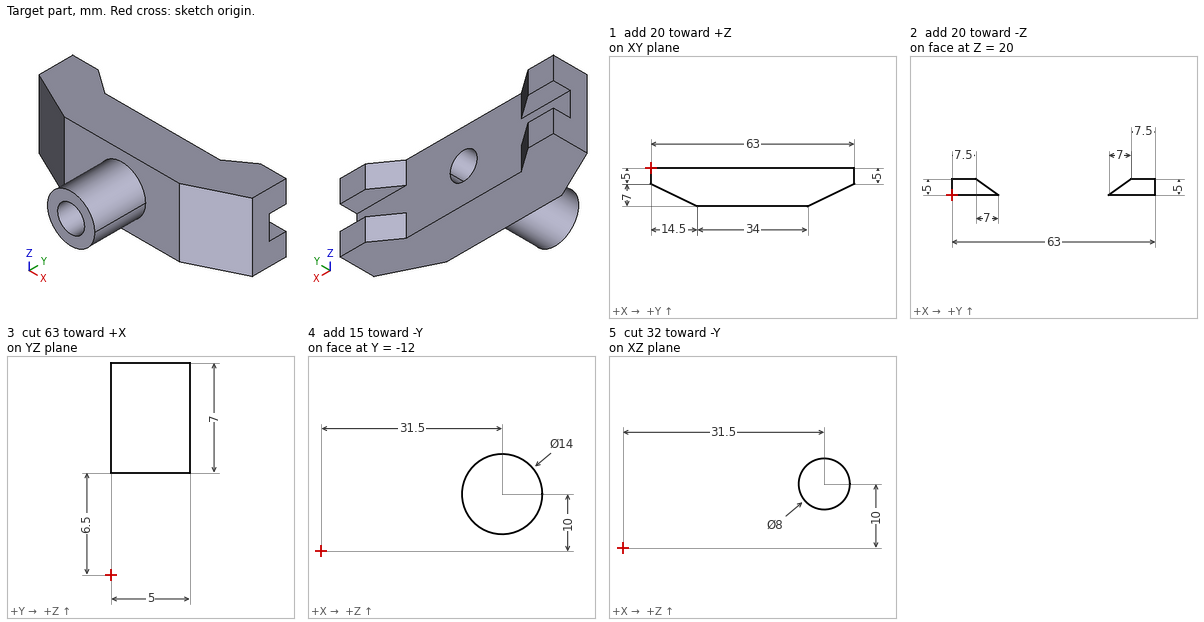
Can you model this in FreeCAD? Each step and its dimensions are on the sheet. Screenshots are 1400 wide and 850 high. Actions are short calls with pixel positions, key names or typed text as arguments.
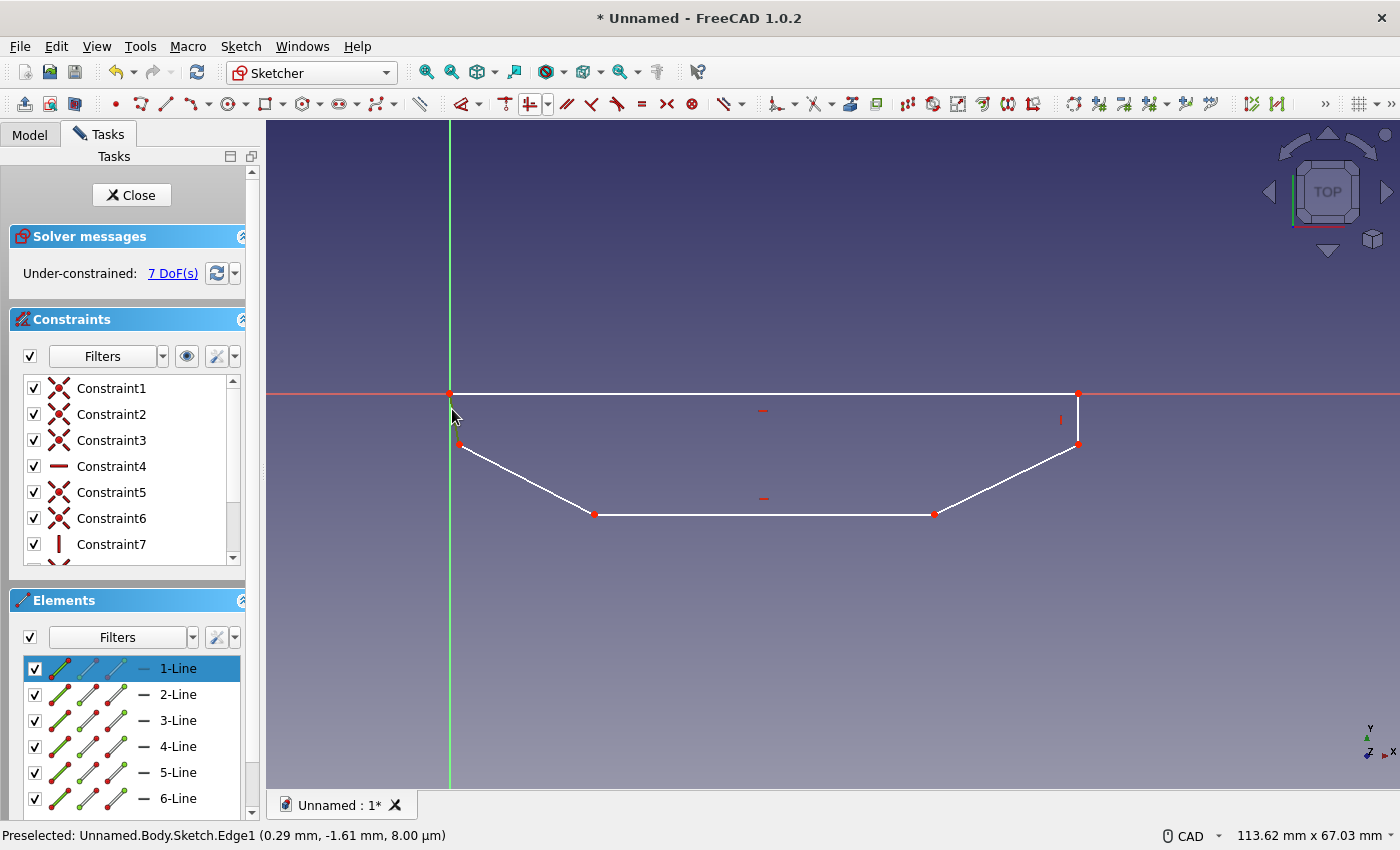
click(548, 104)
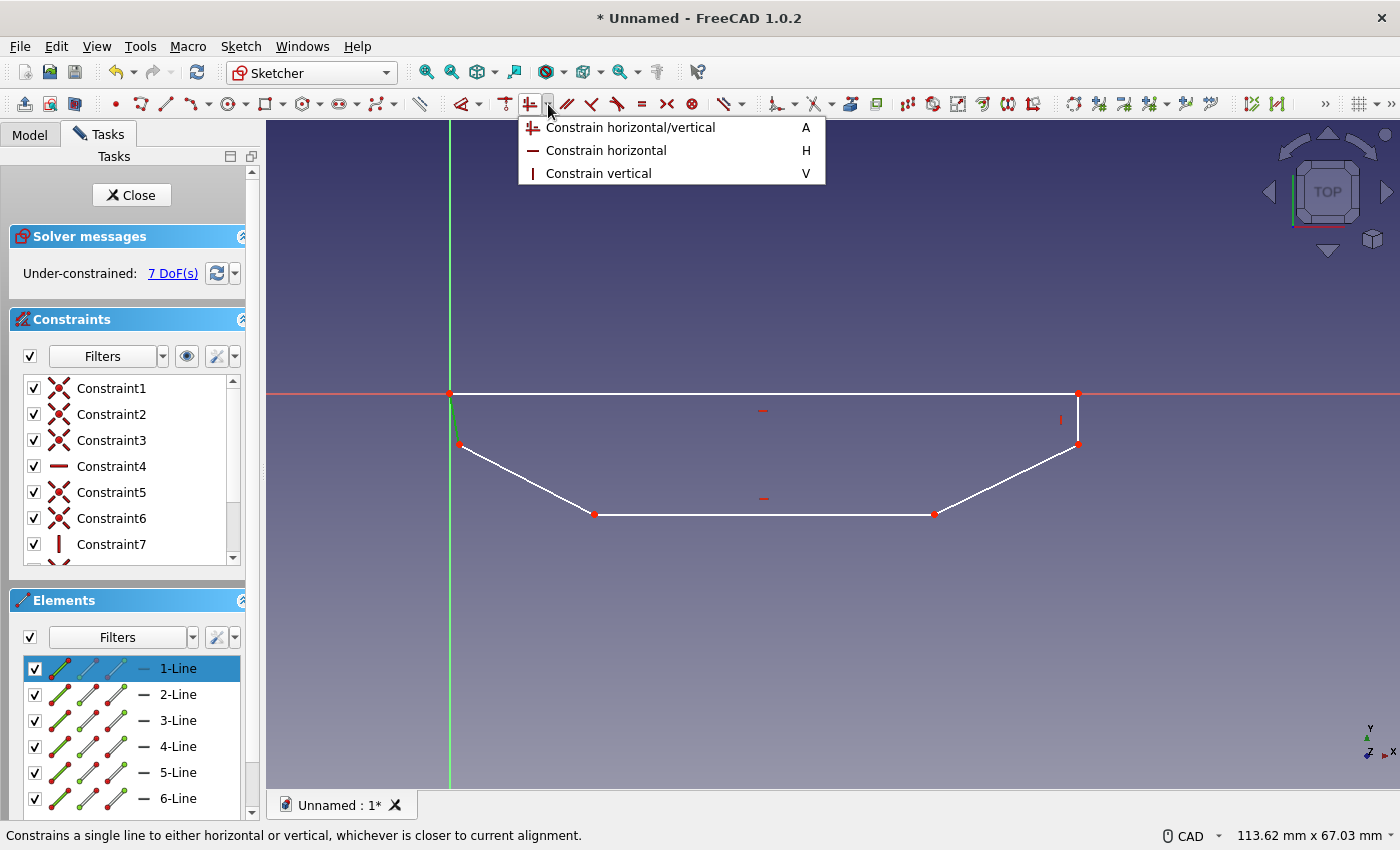
click(672, 174)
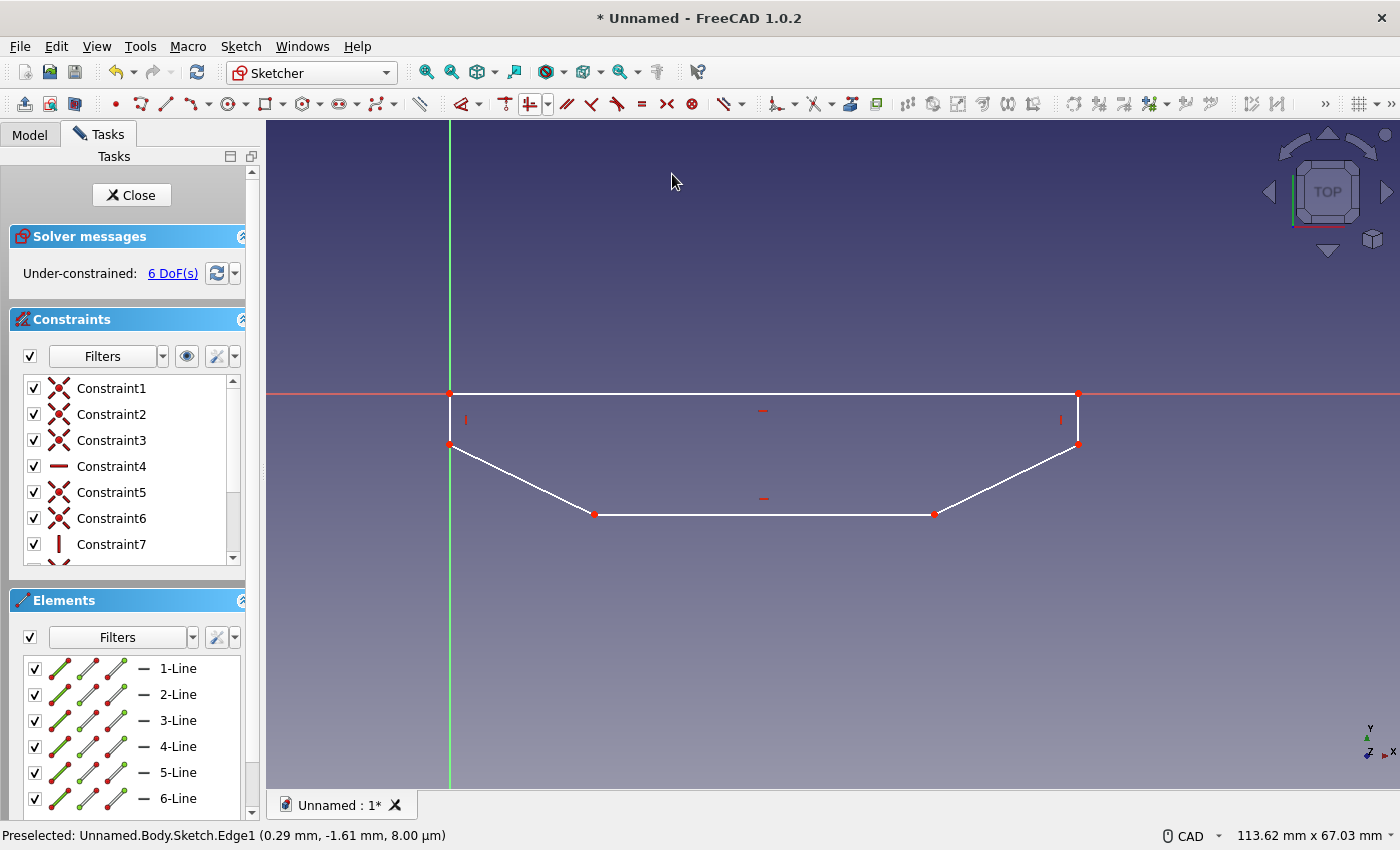
click(460, 104)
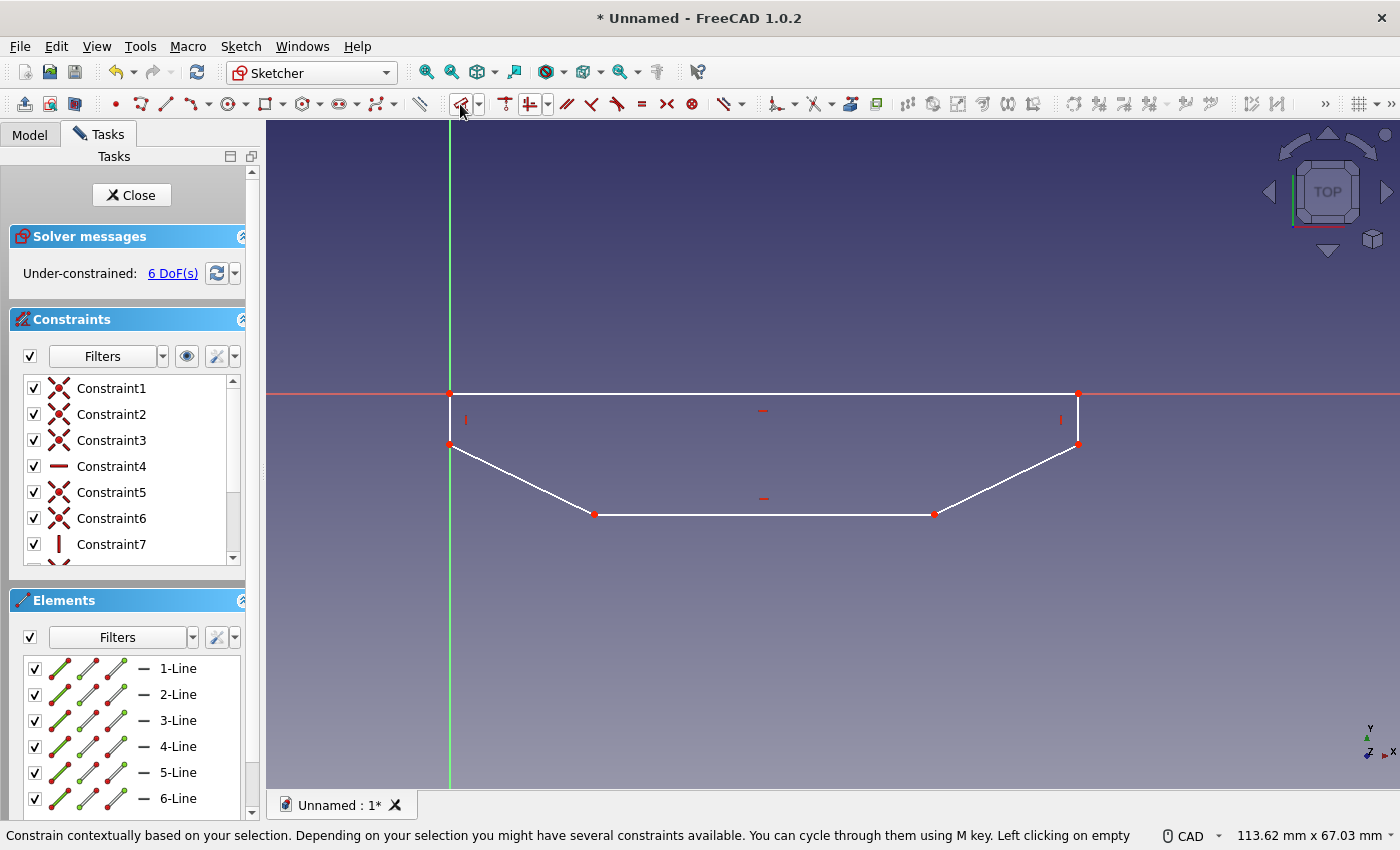
click(450, 409)
click(416, 419)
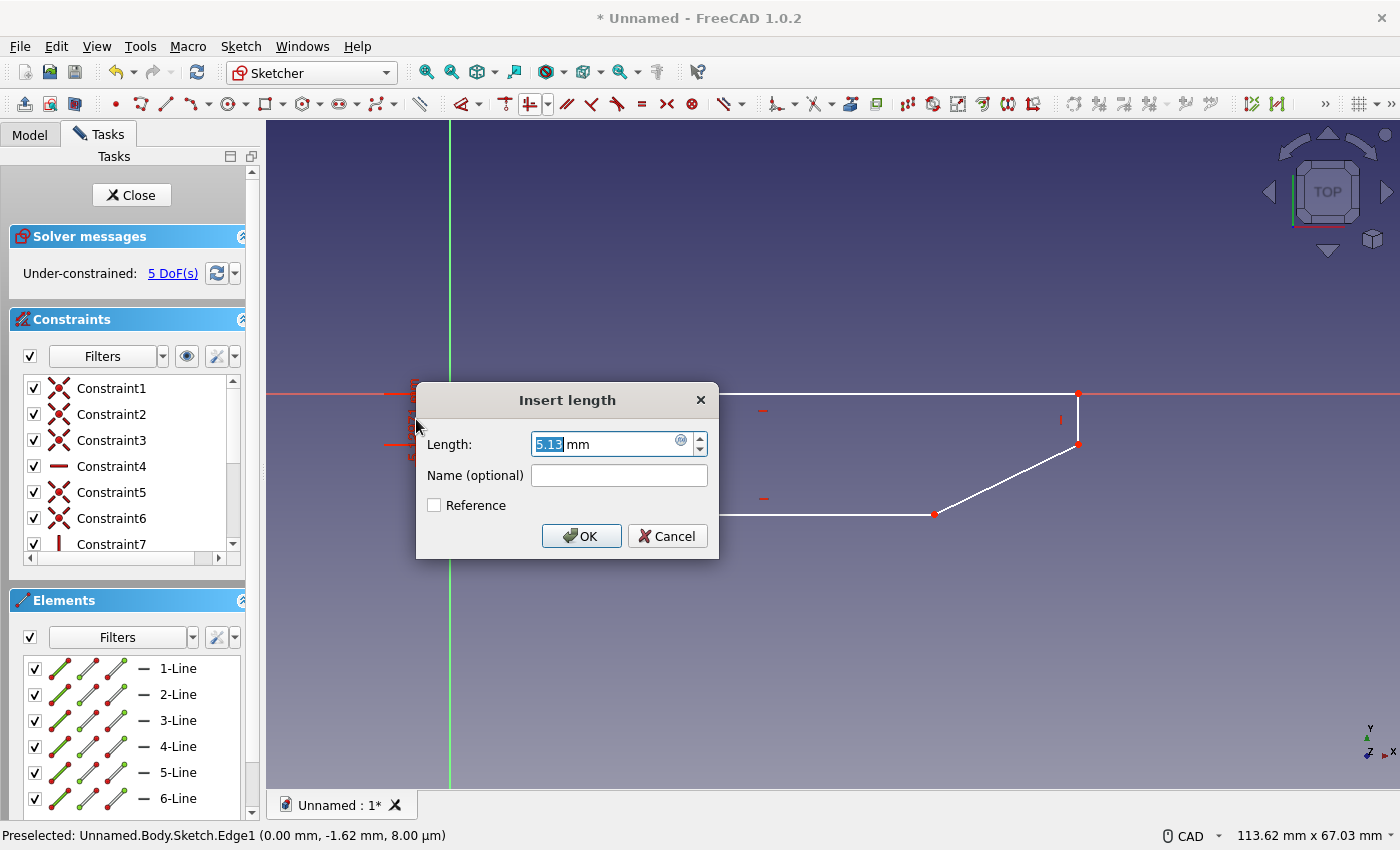
text(5)
key(Return)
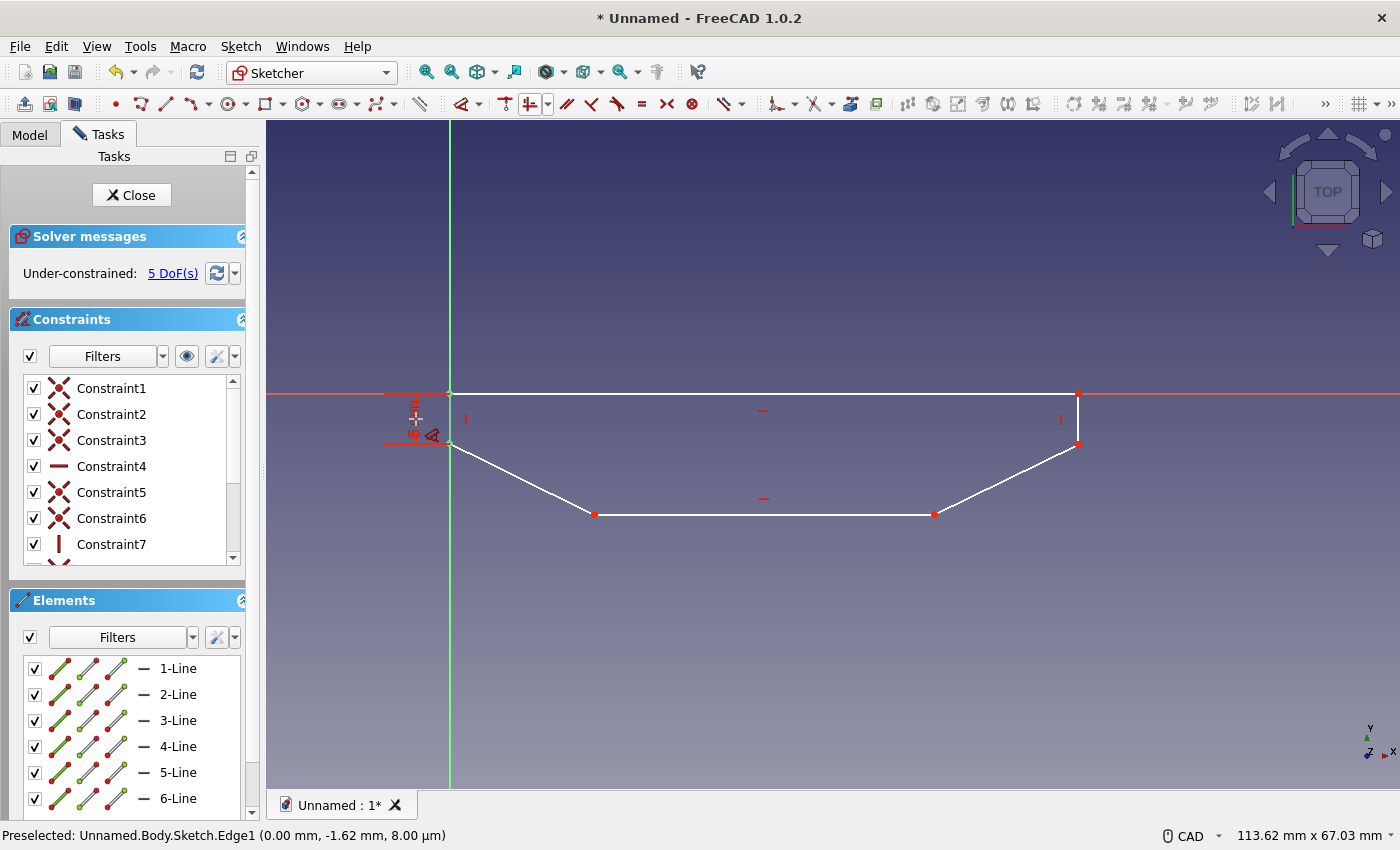
click(1078, 430)
click(1112, 419)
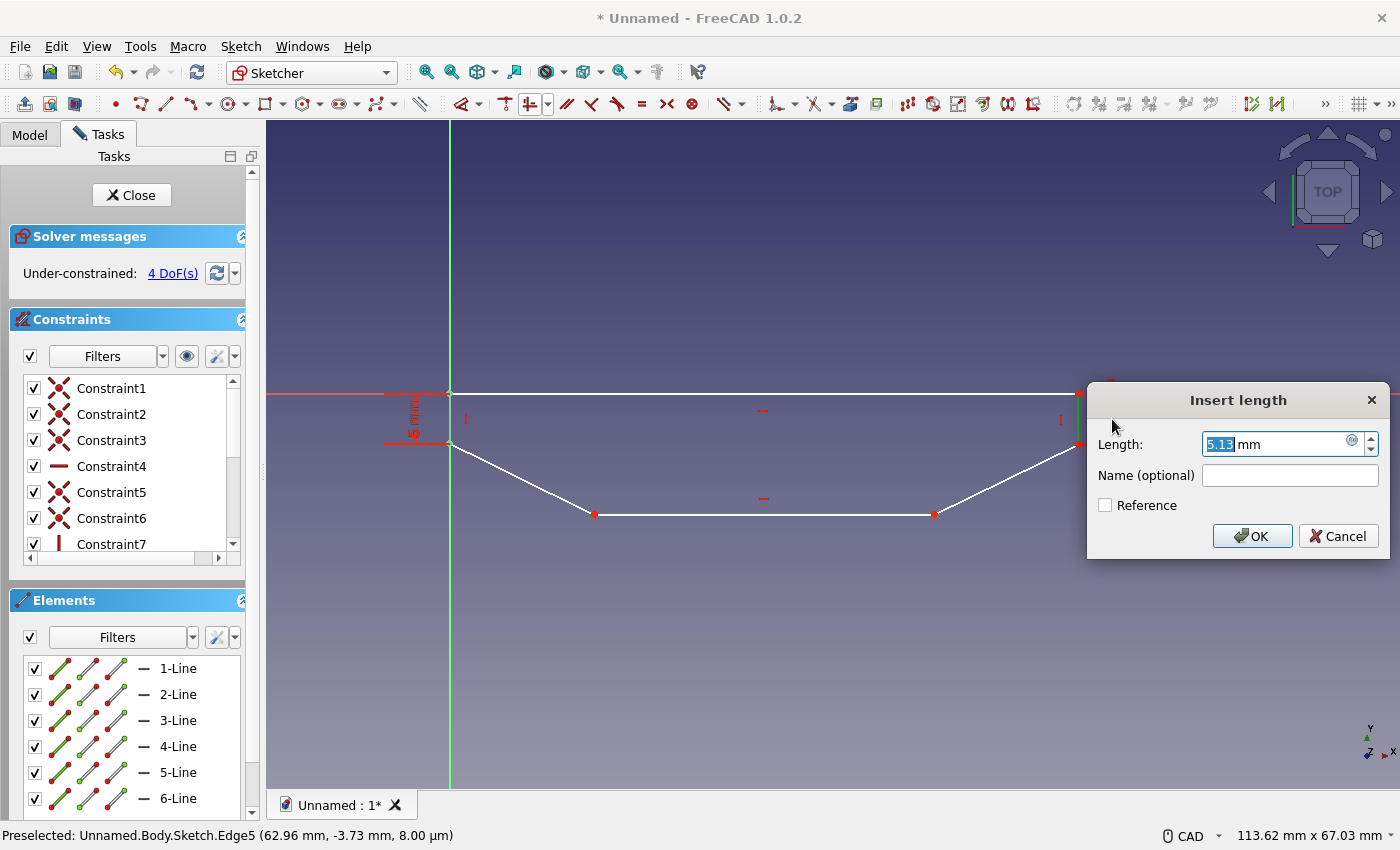
text(5)
key(Return)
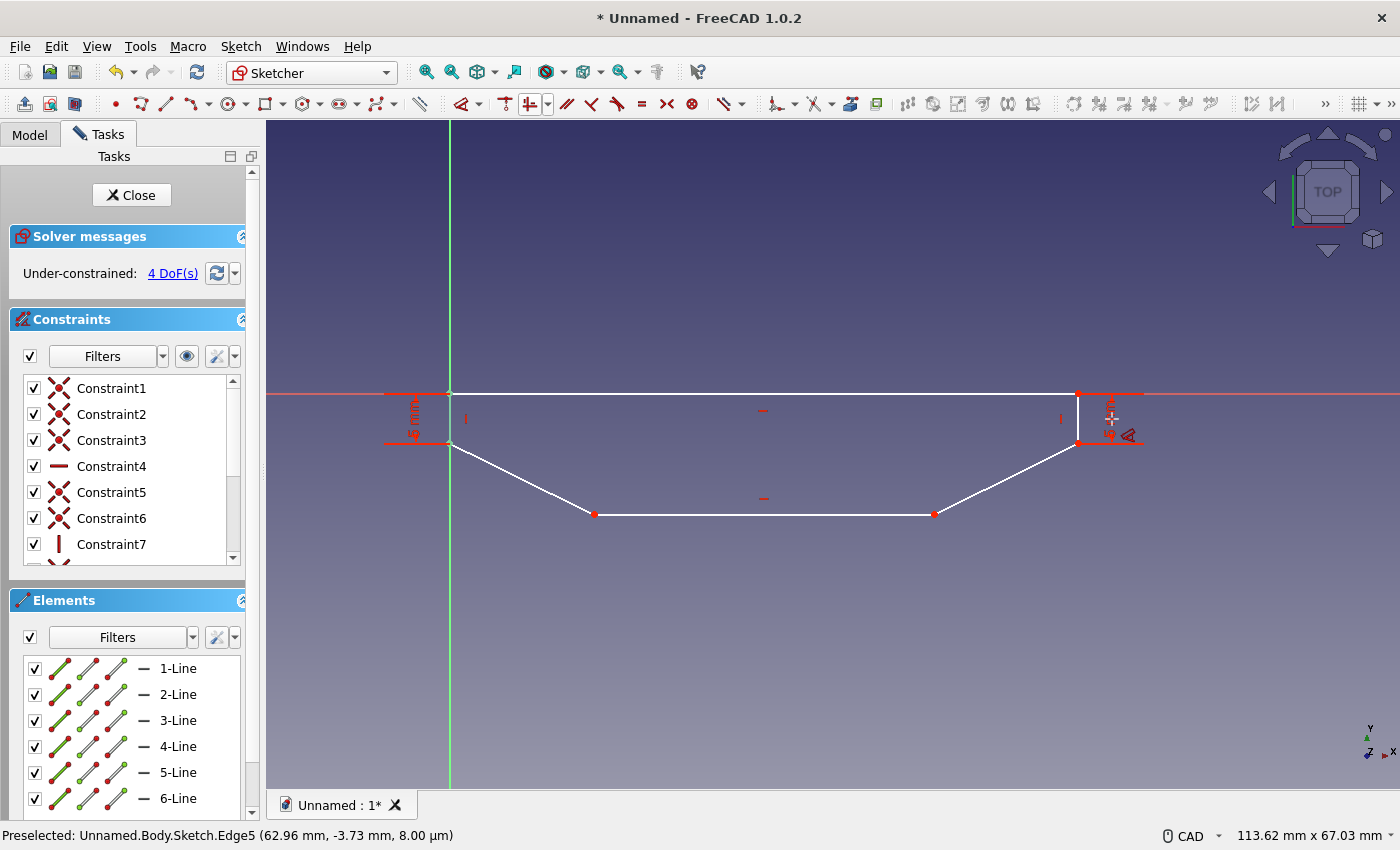
click(696, 515)
click(764, 549)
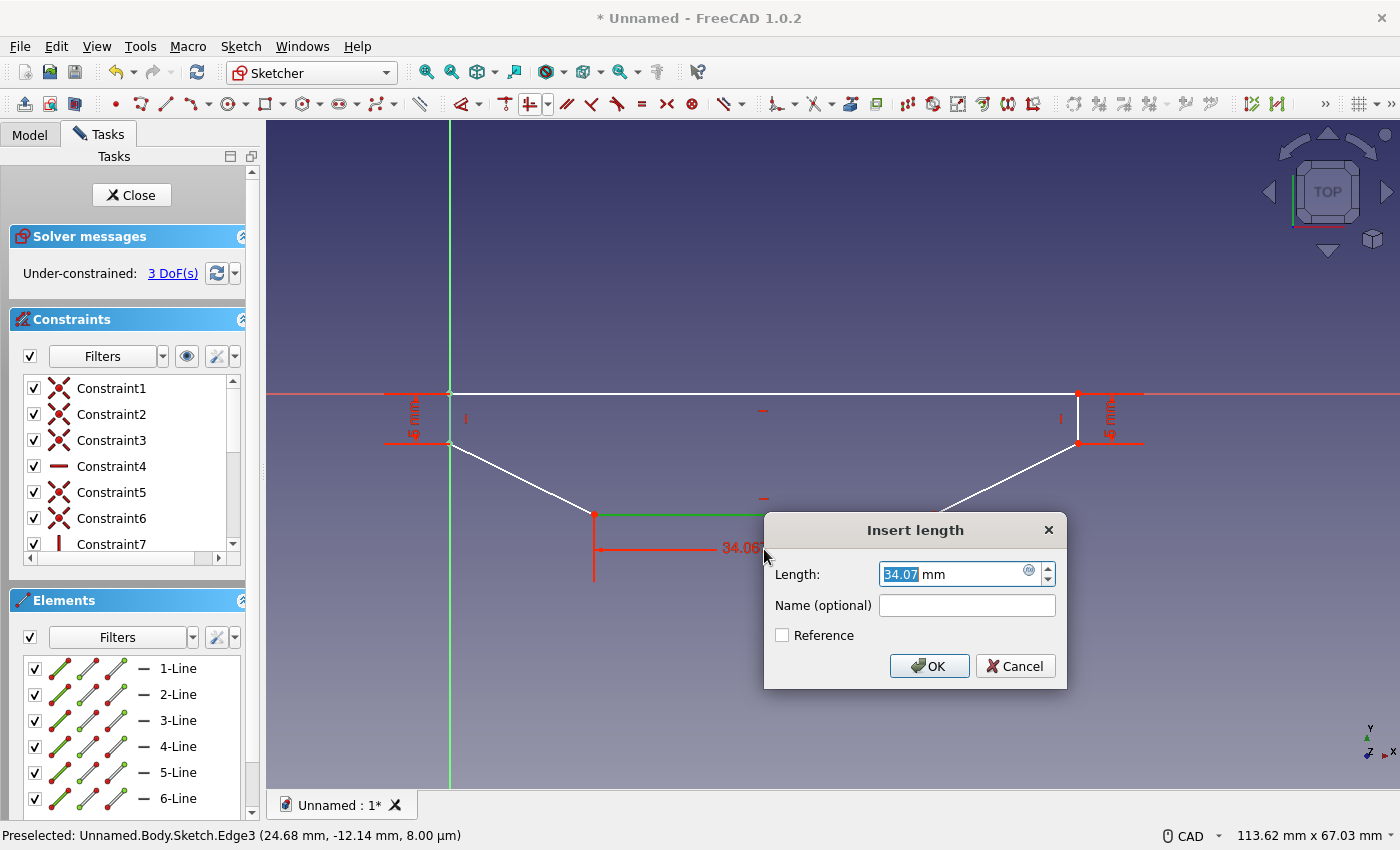
text(34)
key(Return)